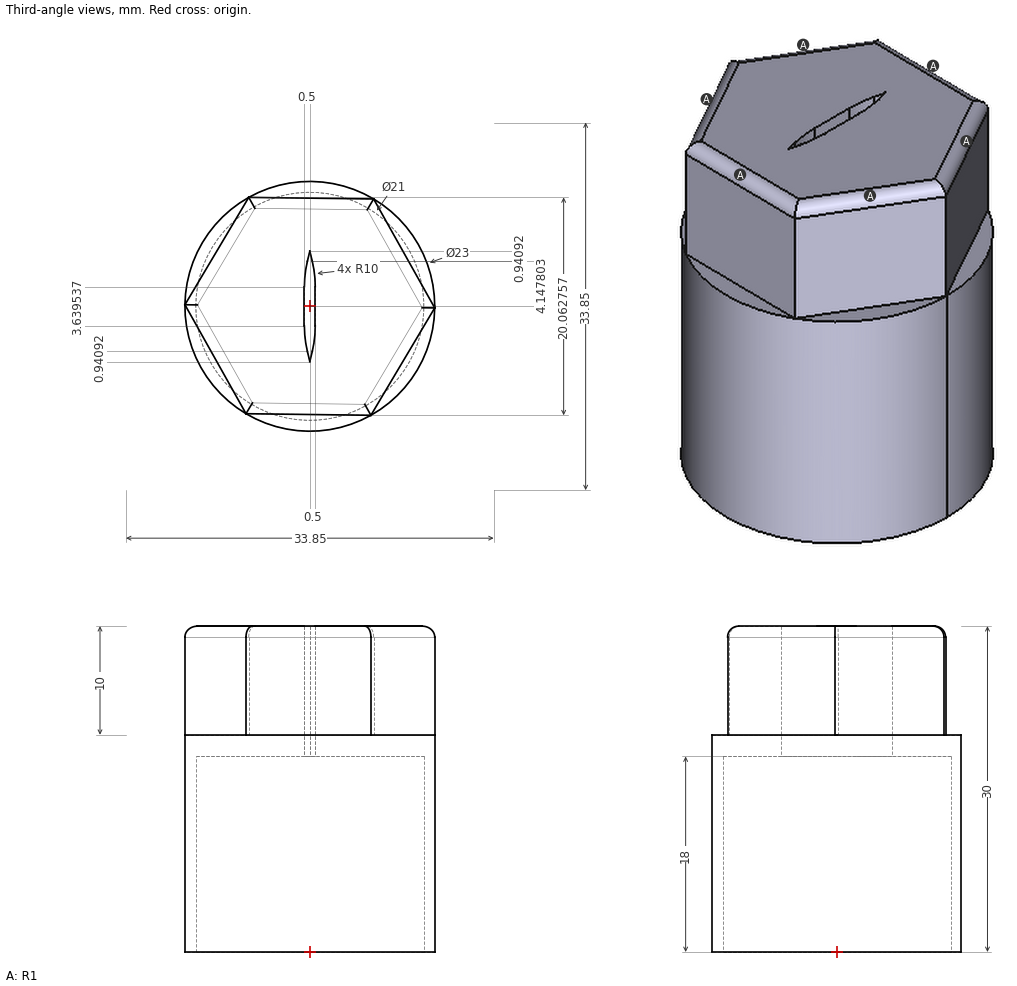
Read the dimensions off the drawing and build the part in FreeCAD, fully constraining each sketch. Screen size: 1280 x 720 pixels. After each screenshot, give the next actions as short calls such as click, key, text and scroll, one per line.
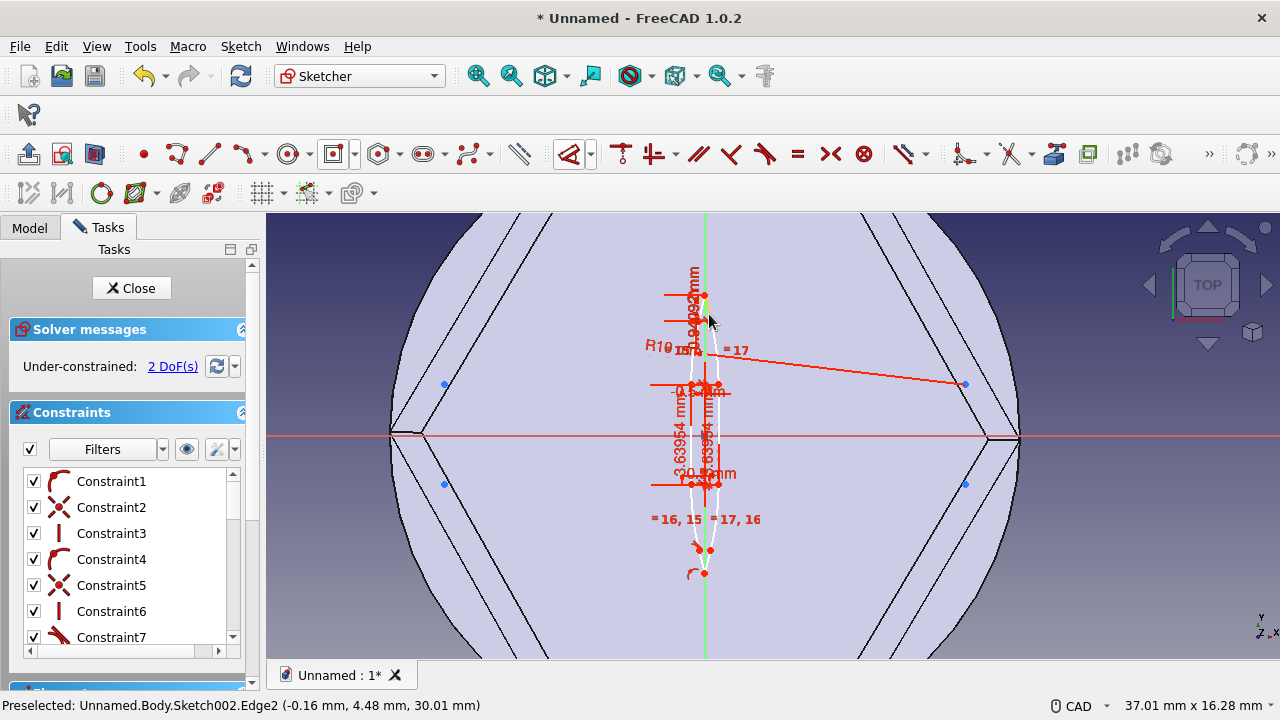
scroll(701, 557, up, 7)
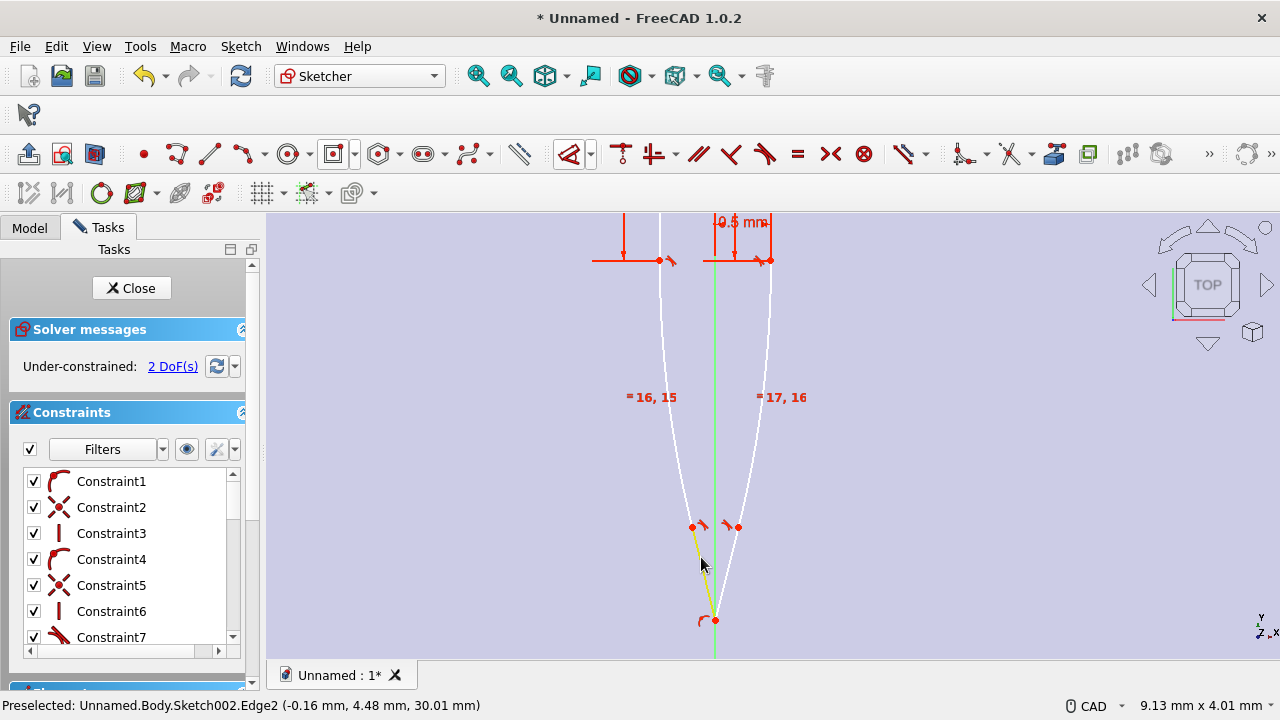
click(699, 555)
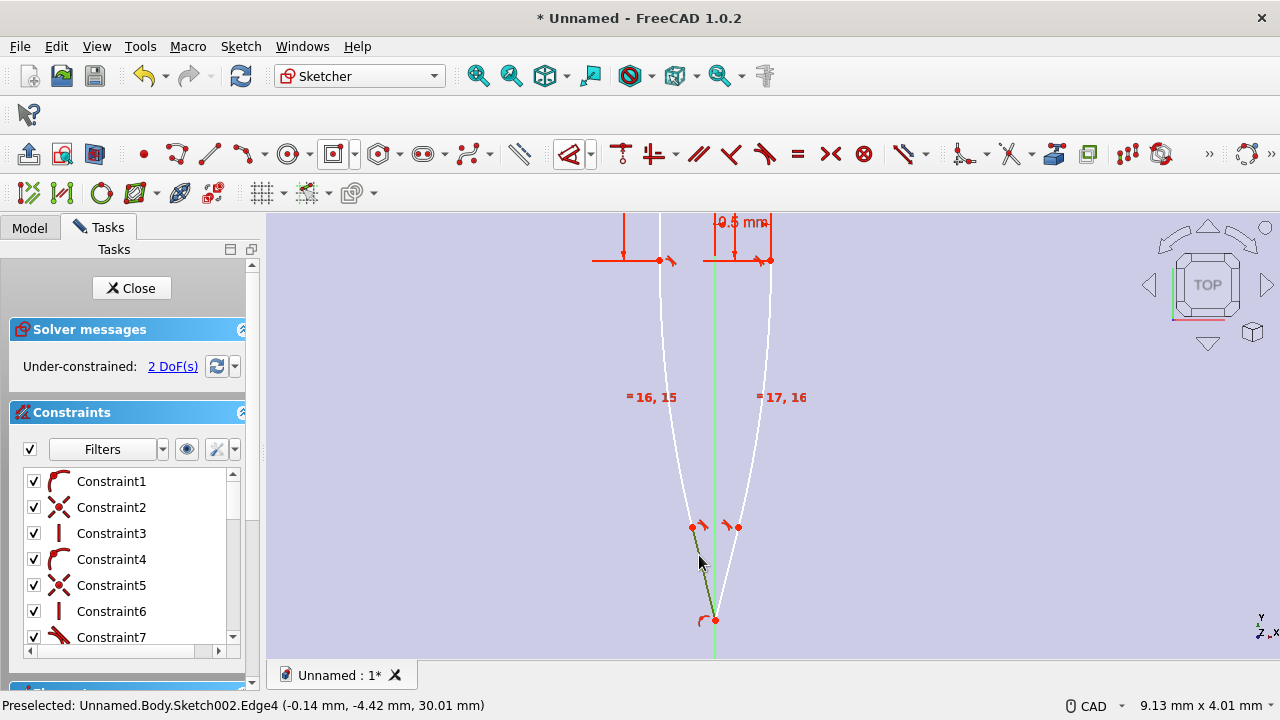
click(590, 154)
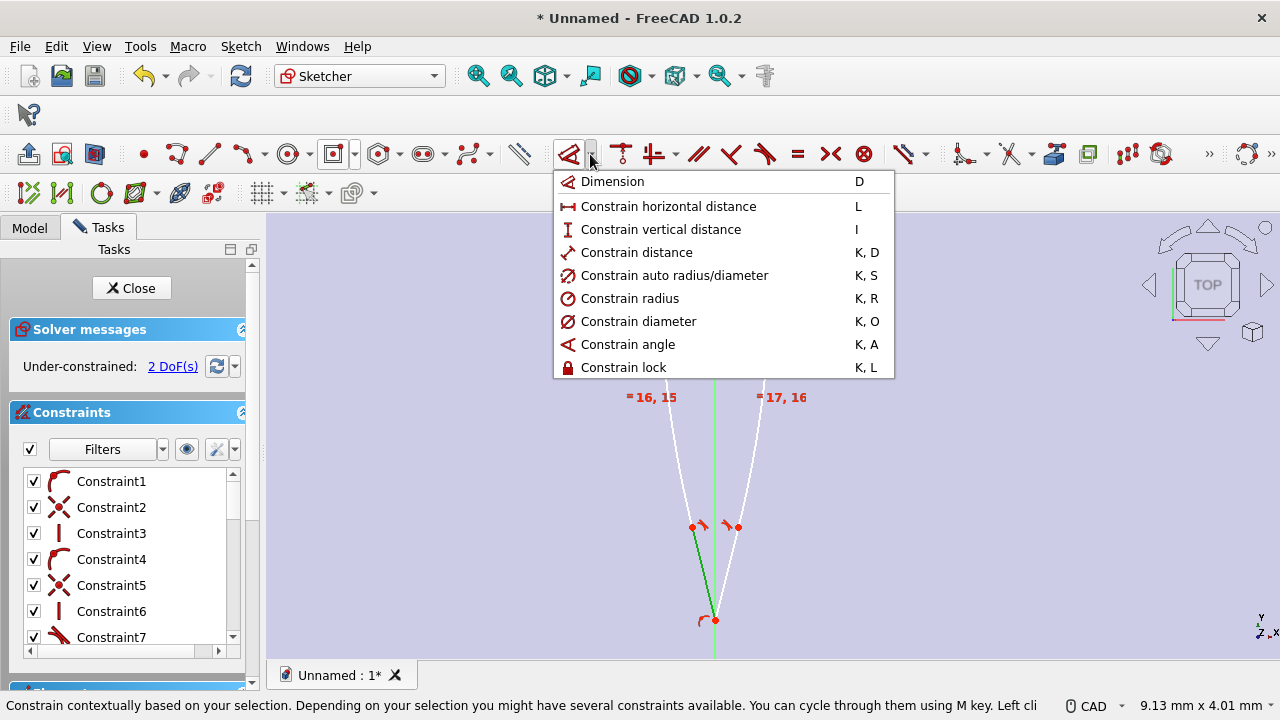
click(724, 230)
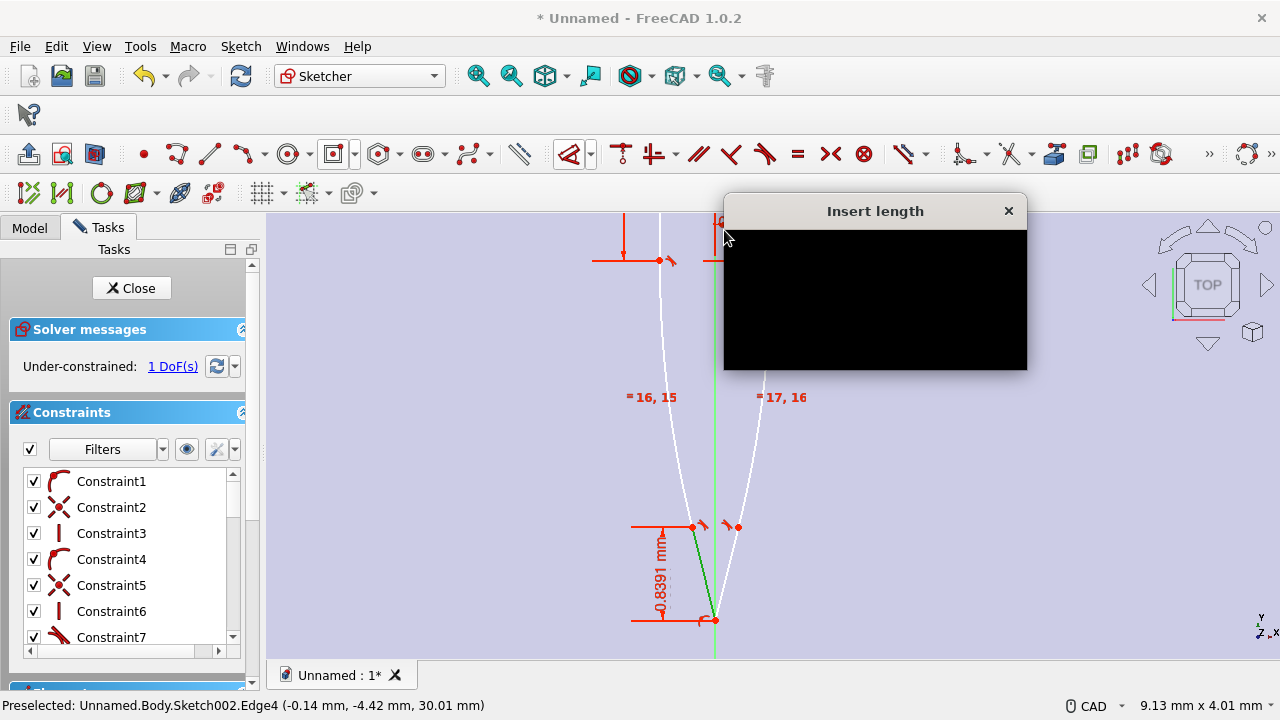
text(0.94092)
key(Return)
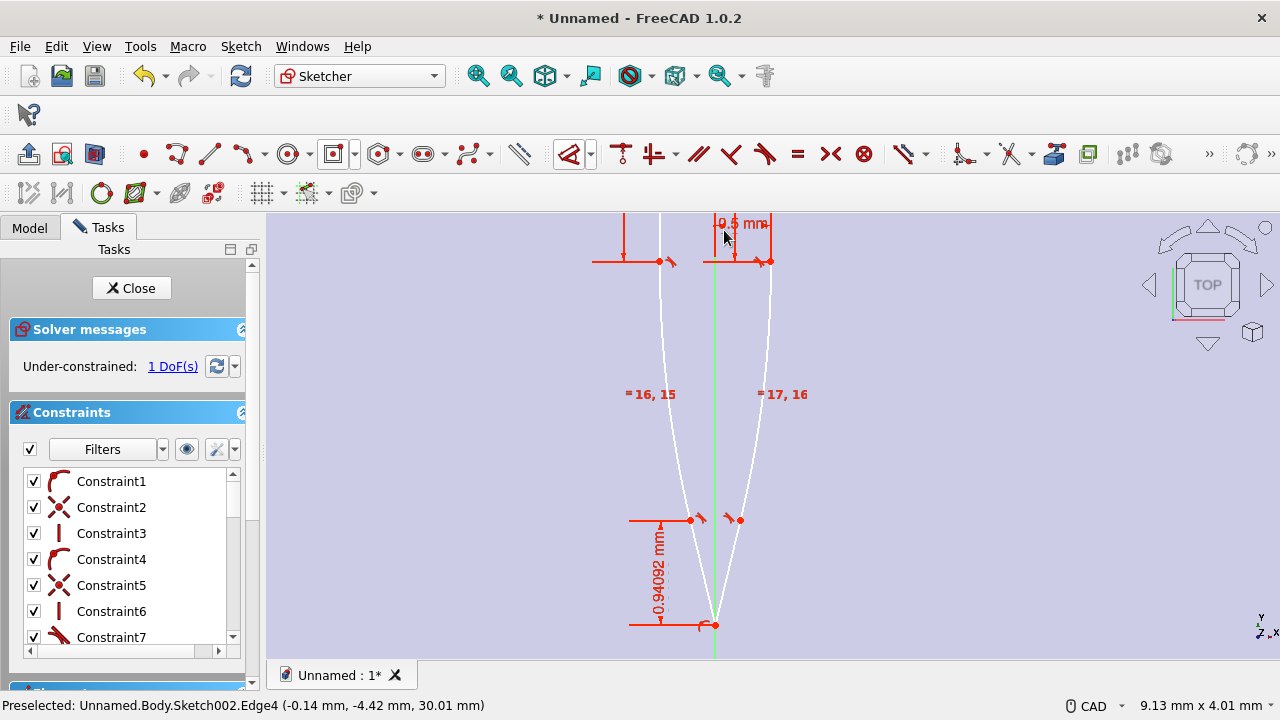
scroll(701, 558, down, 7)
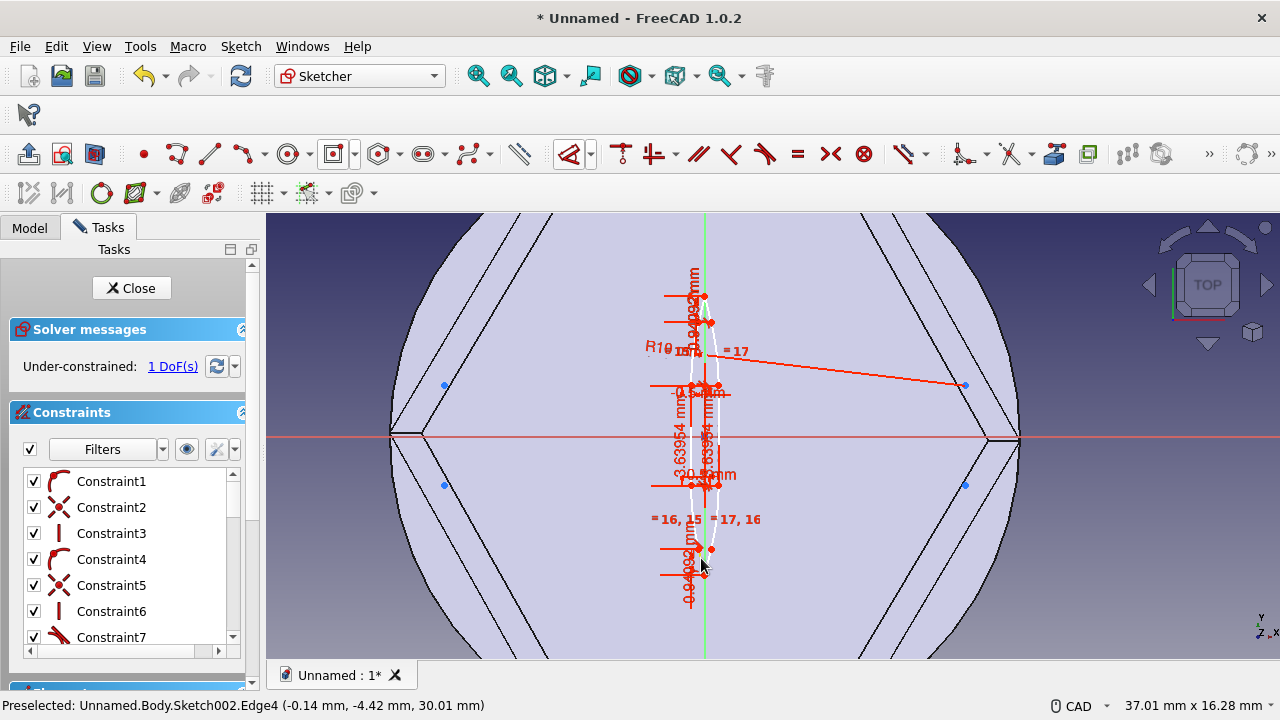
click(711, 322)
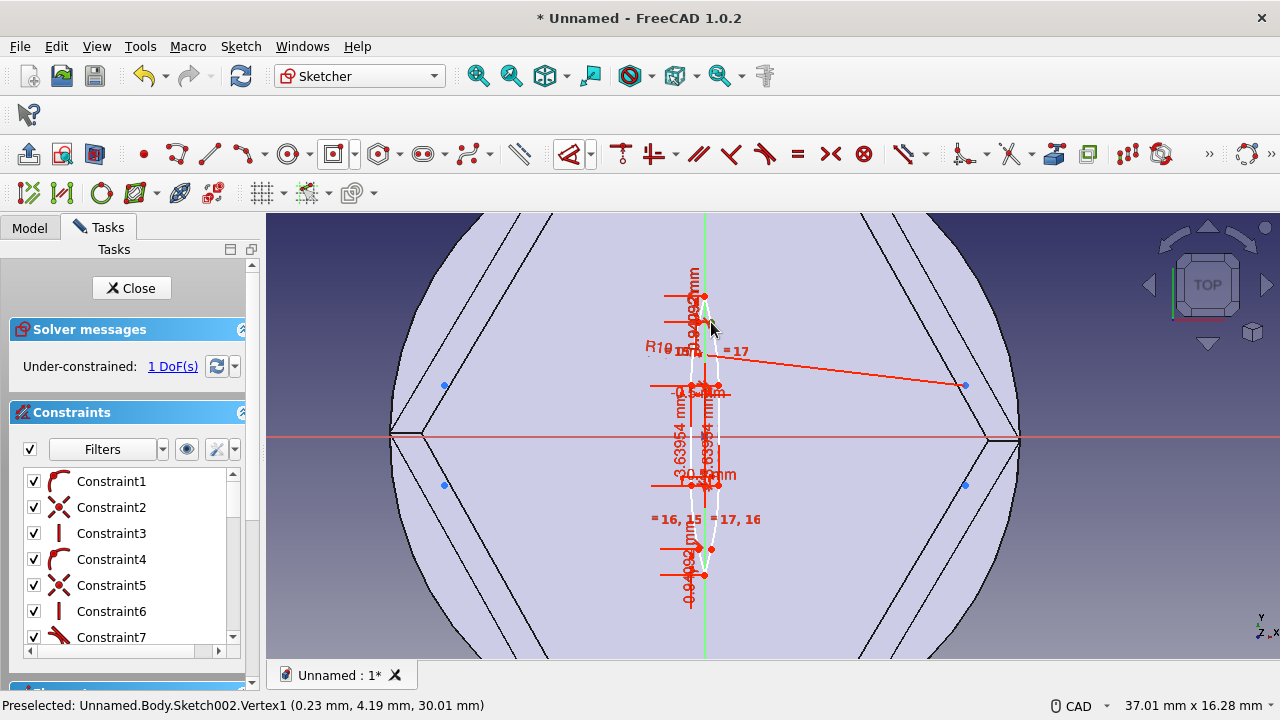
click(590, 154)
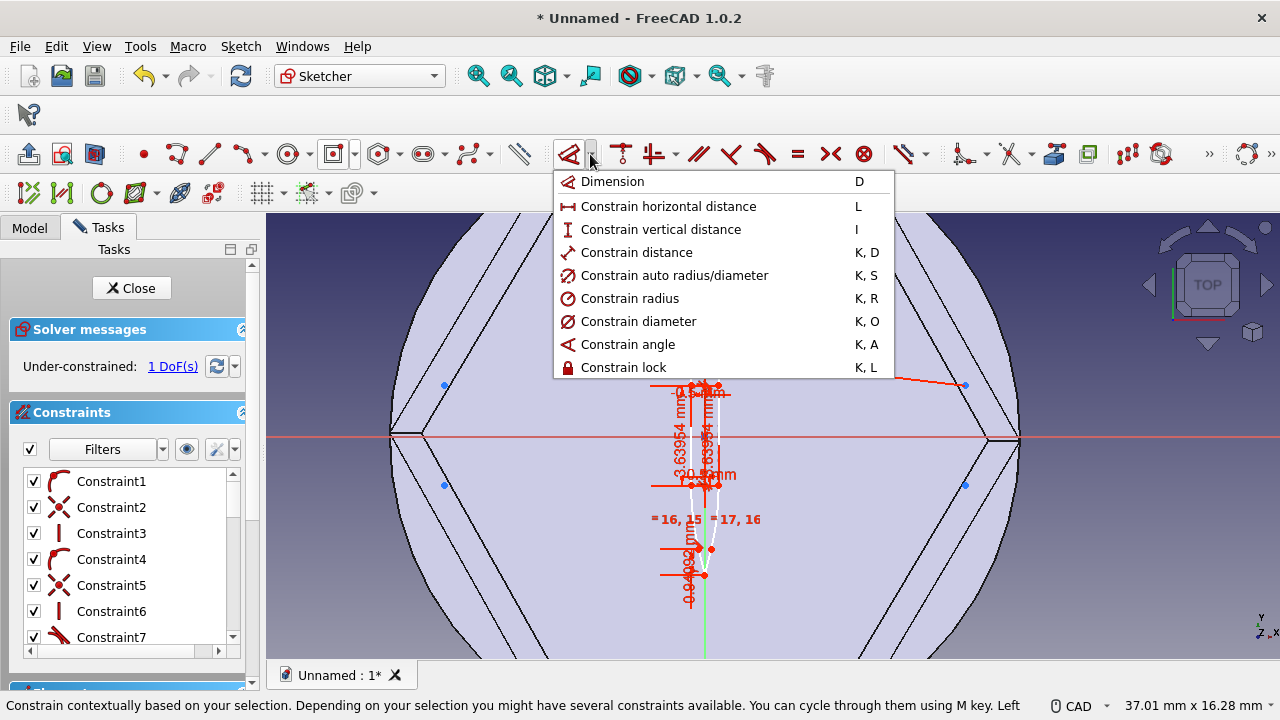
click(724, 230)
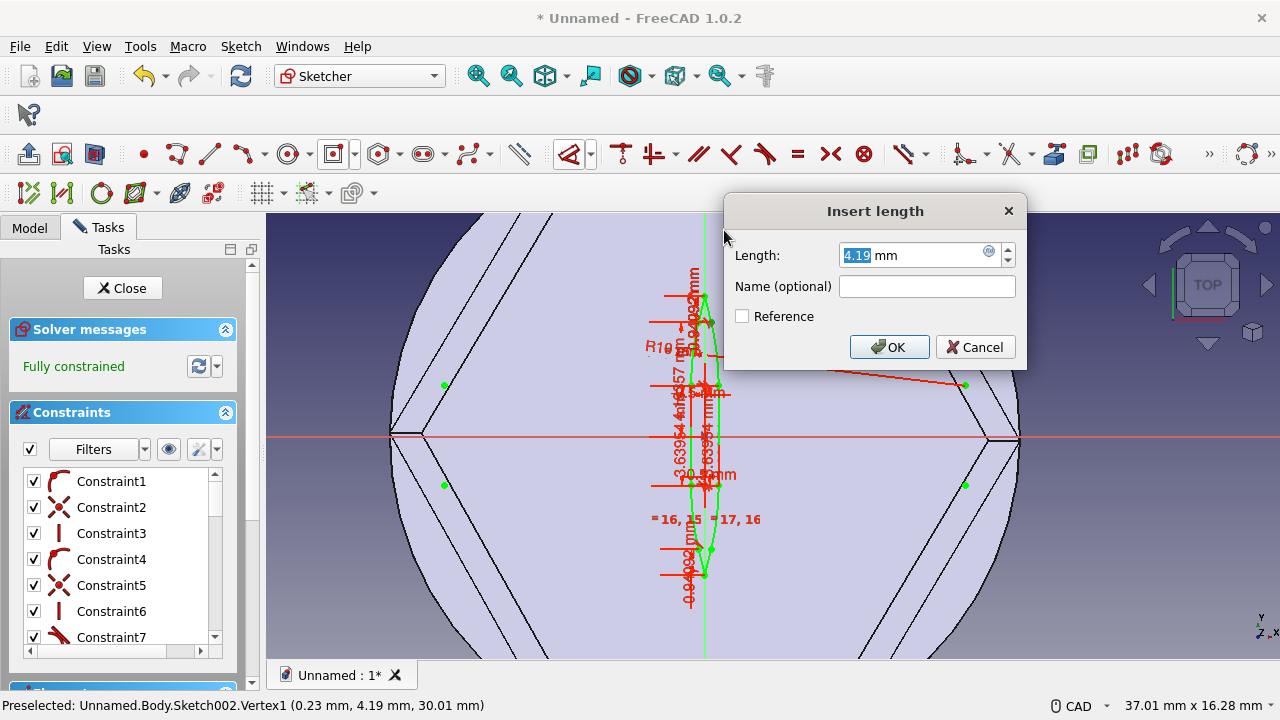
text(4.147803)
key(Return)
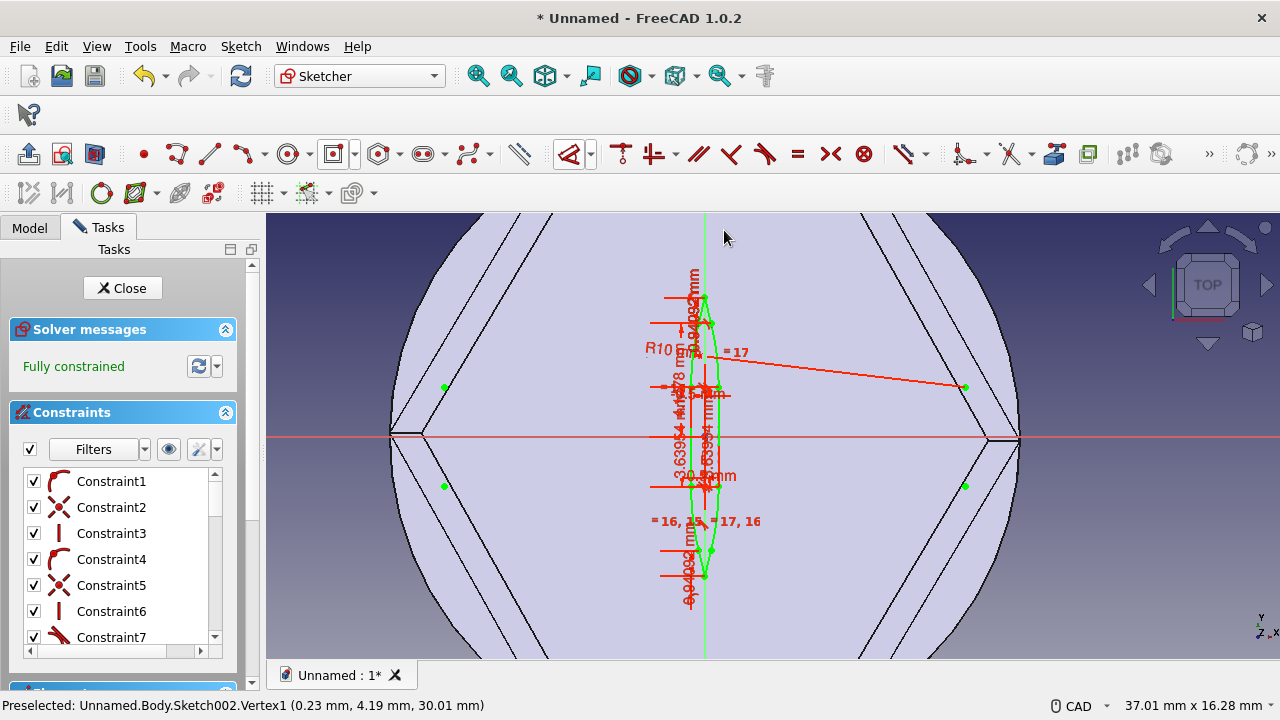
click(123, 288)